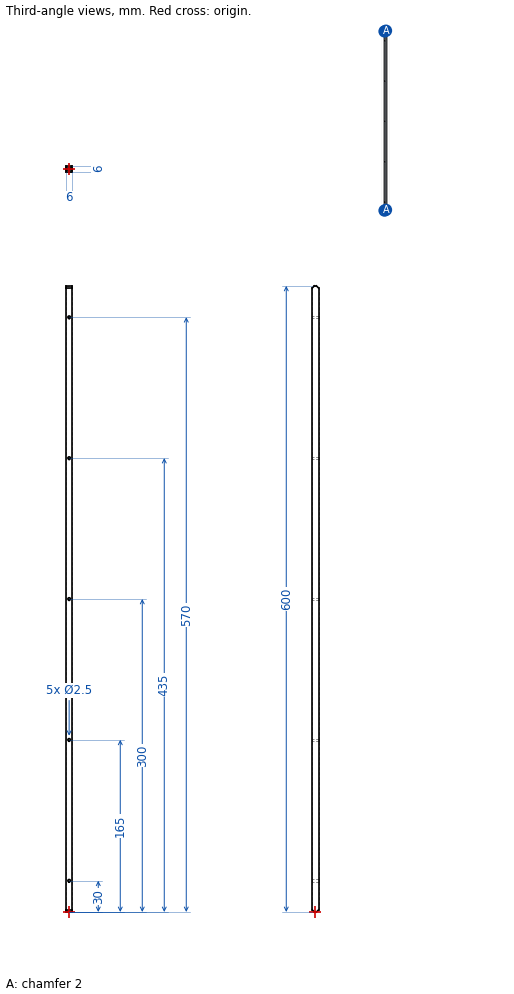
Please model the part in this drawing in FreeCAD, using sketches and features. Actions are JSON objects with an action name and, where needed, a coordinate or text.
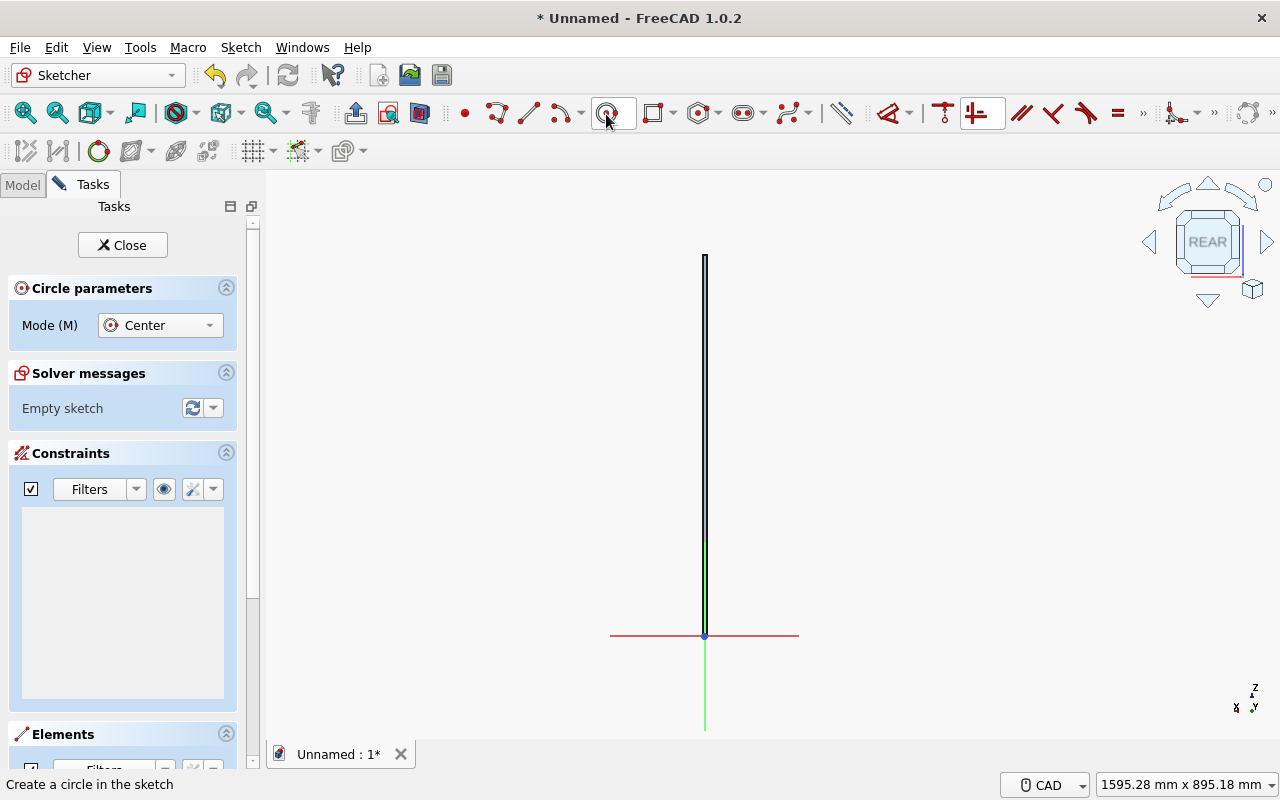
{"action": "scroll", "coordinate": [705, 531], "scroll_direction": "up", "scroll_amount": 17}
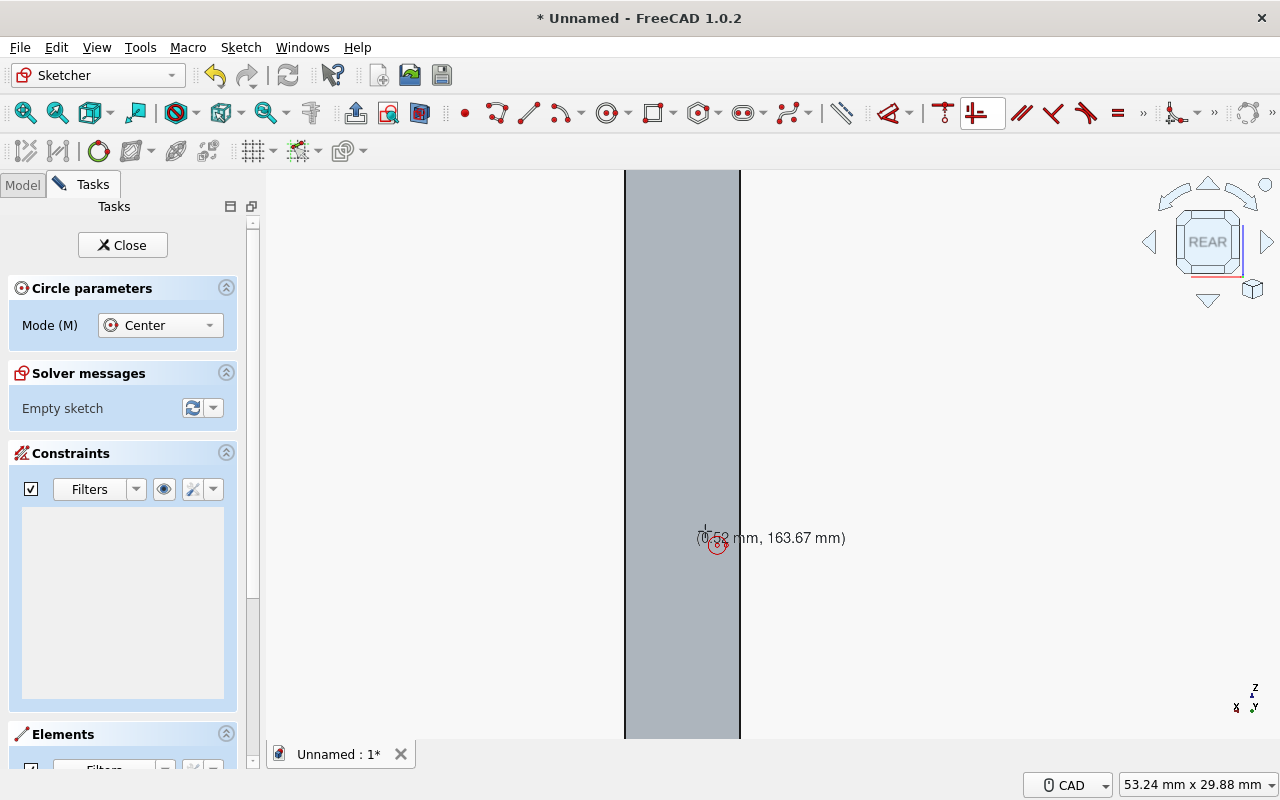
{"action": "scroll", "coordinate": [705, 549], "scroll_direction": "down", "scroll_amount": 16}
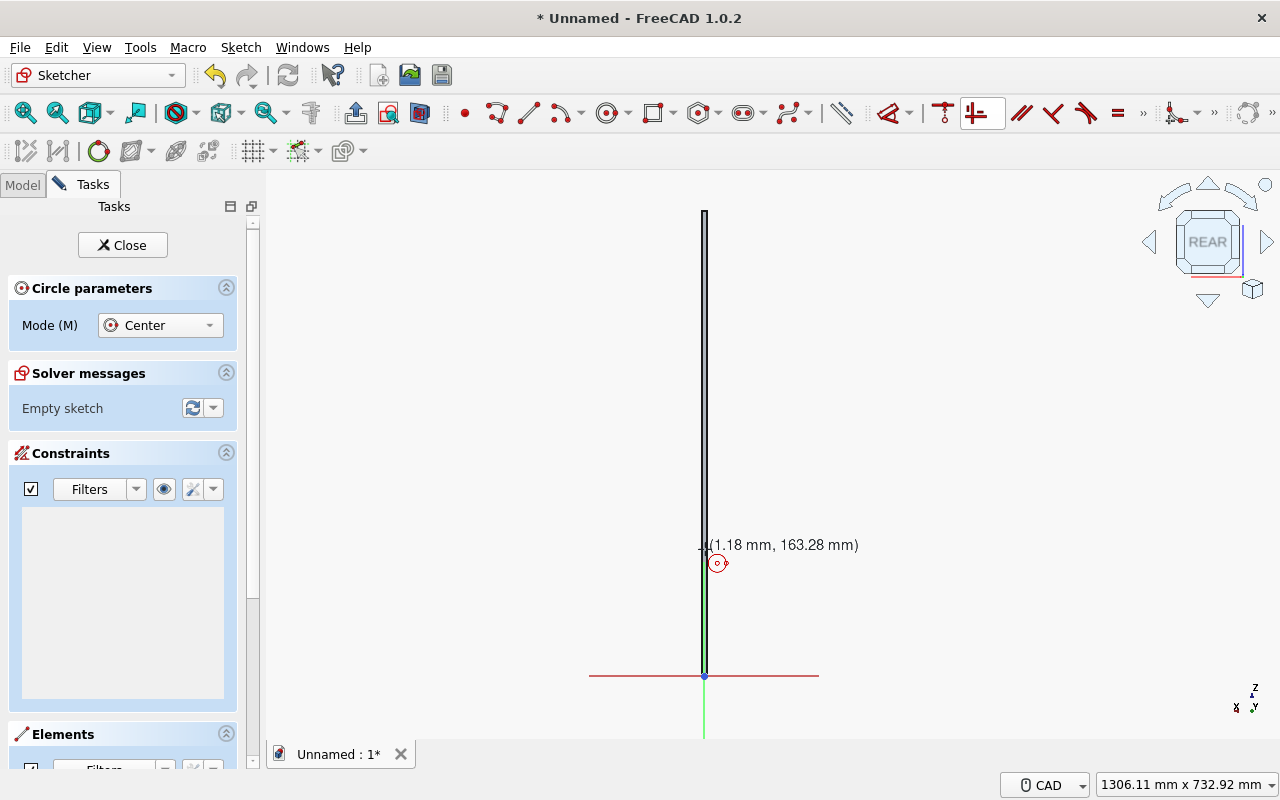
{"action": "left_click", "coordinate": [704, 548]}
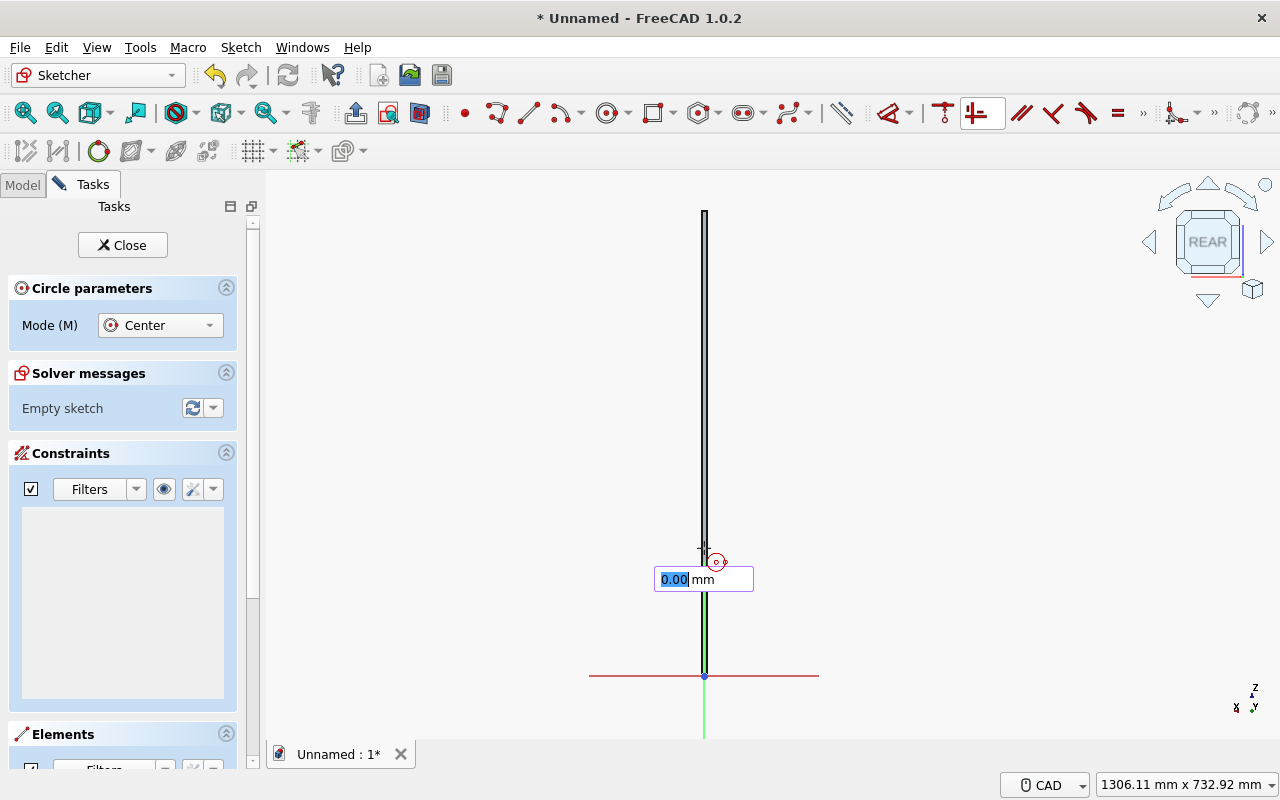
{"action": "scroll", "coordinate": [705, 548], "scroll_direction": "up", "scroll_amount": 15}
{"action": "mouse_move", "coordinate": [705, 536]}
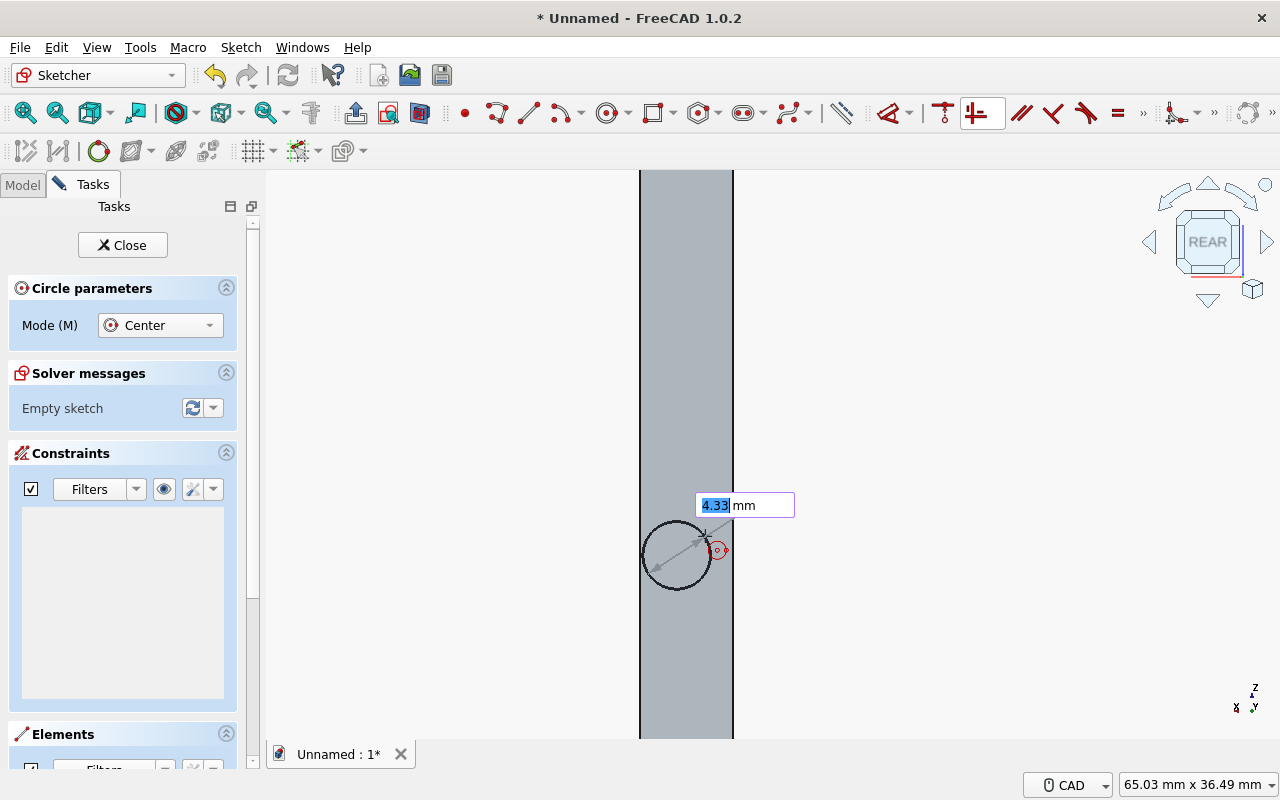
{"action": "type", "text": "2.5"}
{"action": "key", "text": "Return"}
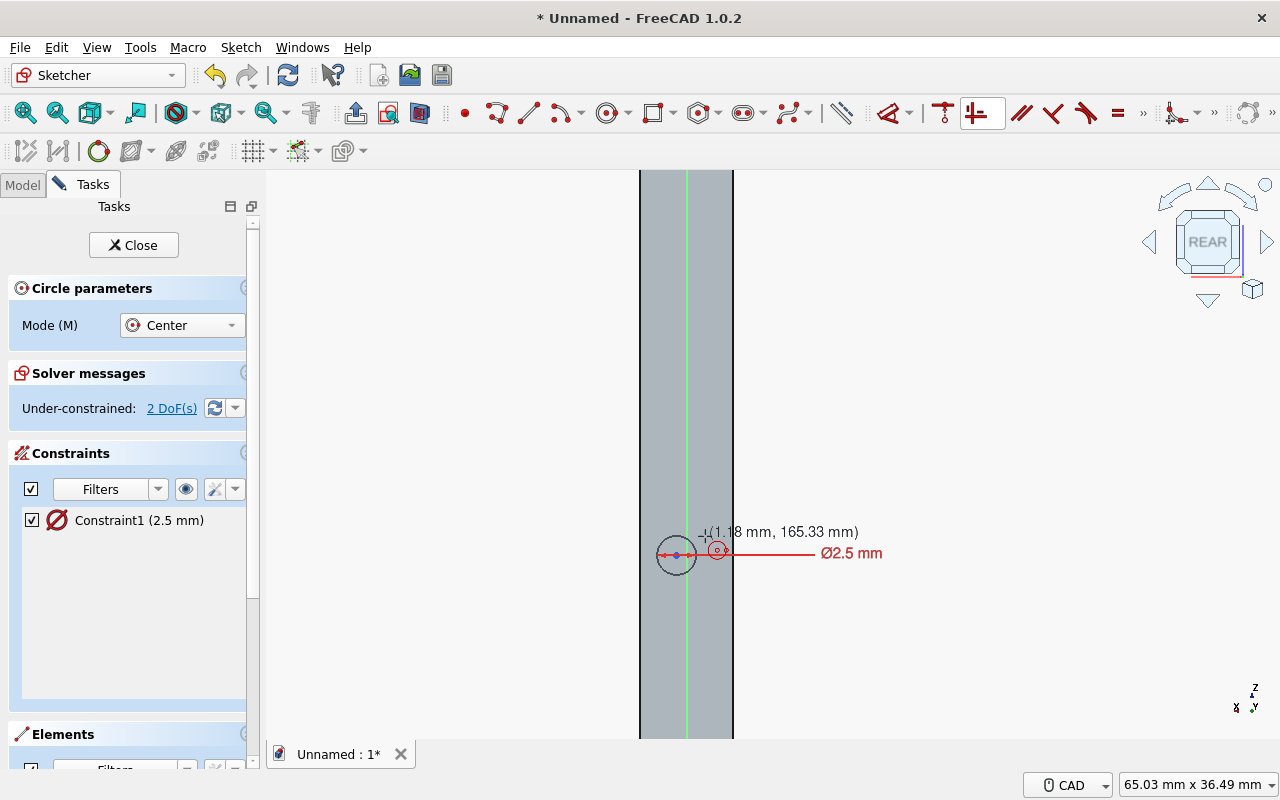
{"action": "scroll", "coordinate": [705, 548], "scroll_direction": "down", "scroll_amount": 15}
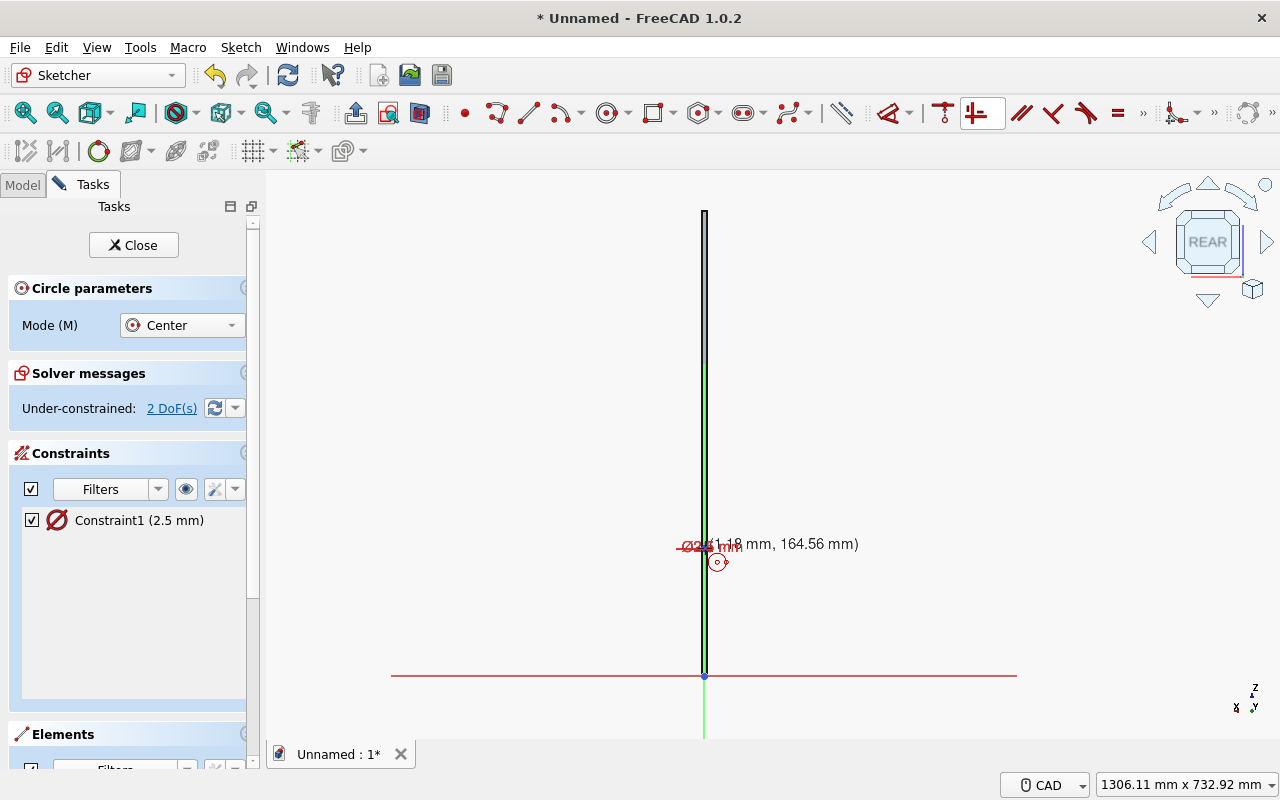
{"action": "scroll", "coordinate": [704, 444], "scroll_direction": "up", "scroll_amount": 16}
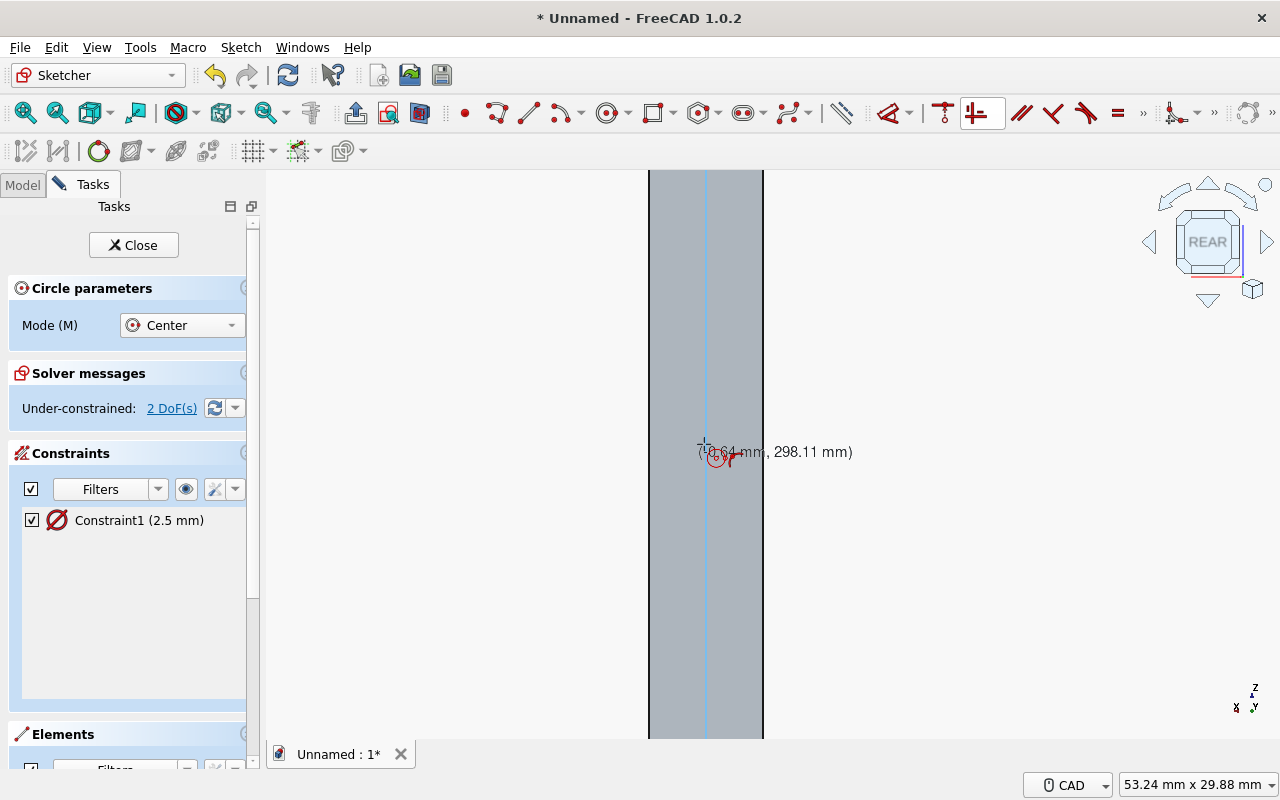
{"action": "scroll", "coordinate": [704, 444], "scroll_direction": "down", "scroll_amount": 16}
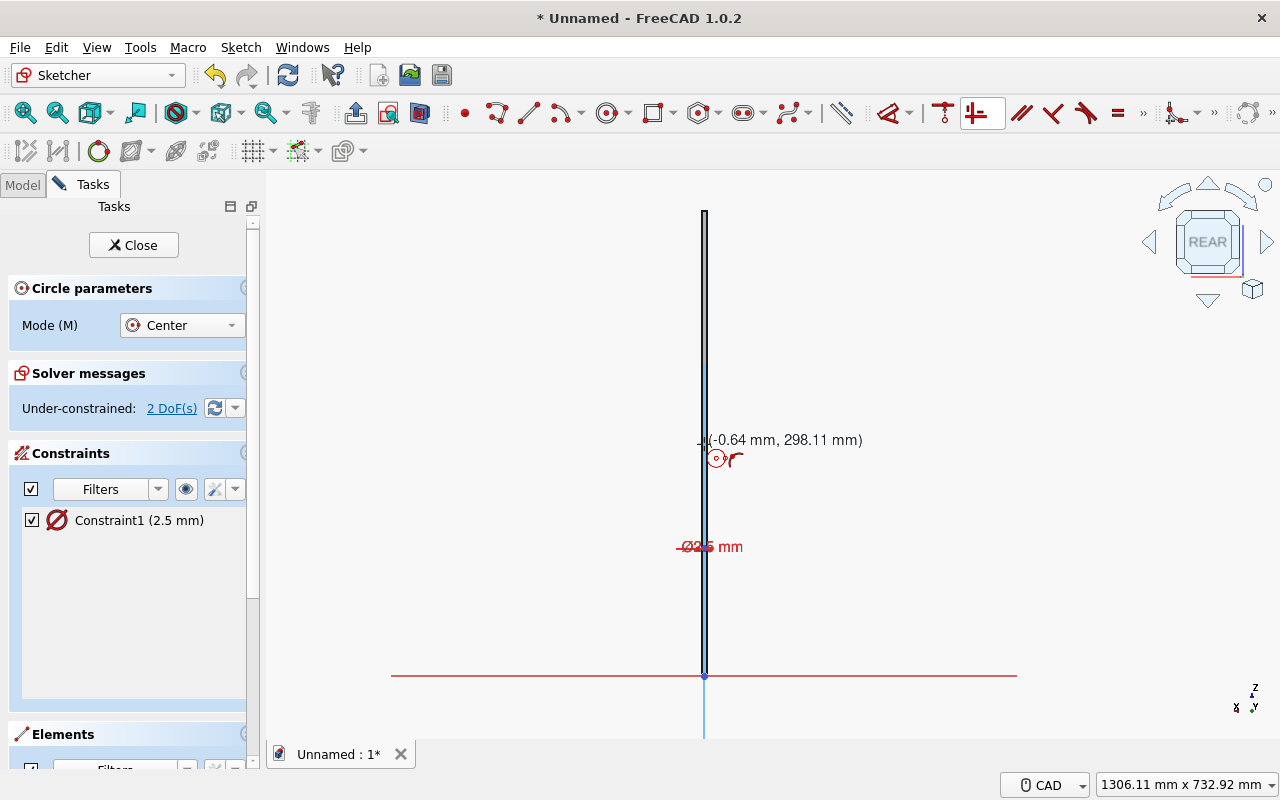
{"action": "left_click", "coordinate": [704, 444]}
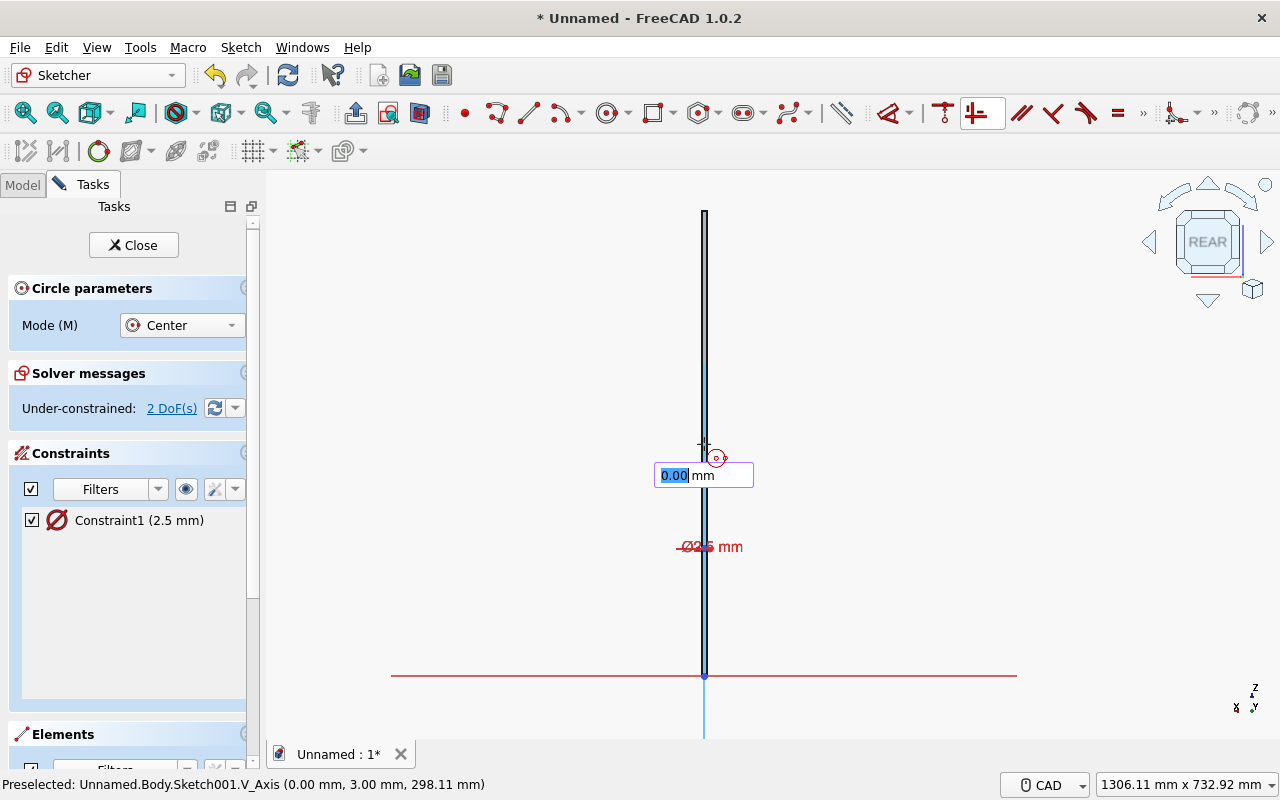
{"action": "scroll", "coordinate": [705, 443], "scroll_direction": "up", "scroll_amount": 15}
{"action": "mouse_move", "coordinate": [705, 438]}